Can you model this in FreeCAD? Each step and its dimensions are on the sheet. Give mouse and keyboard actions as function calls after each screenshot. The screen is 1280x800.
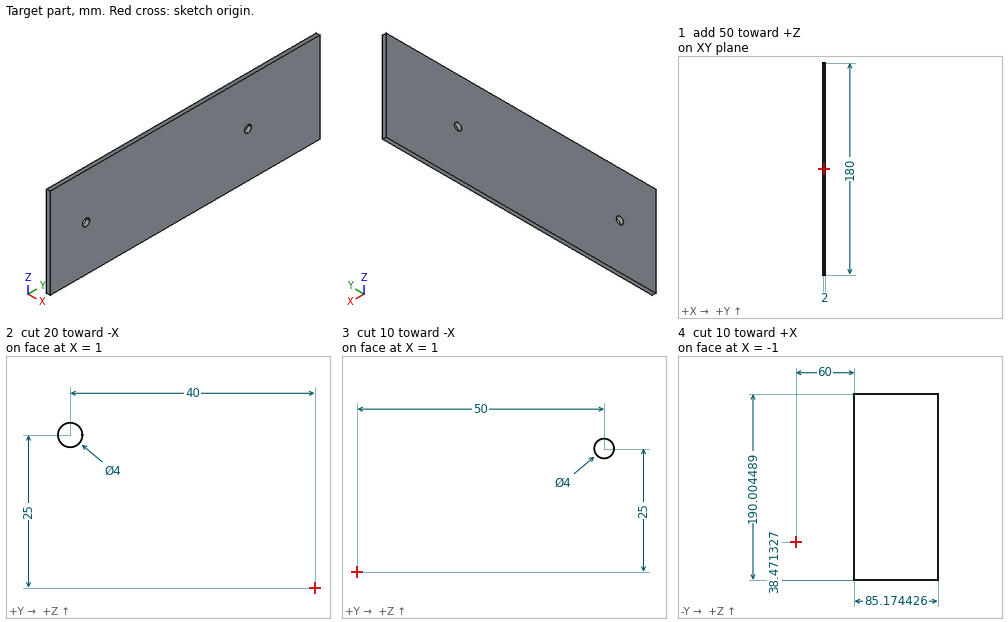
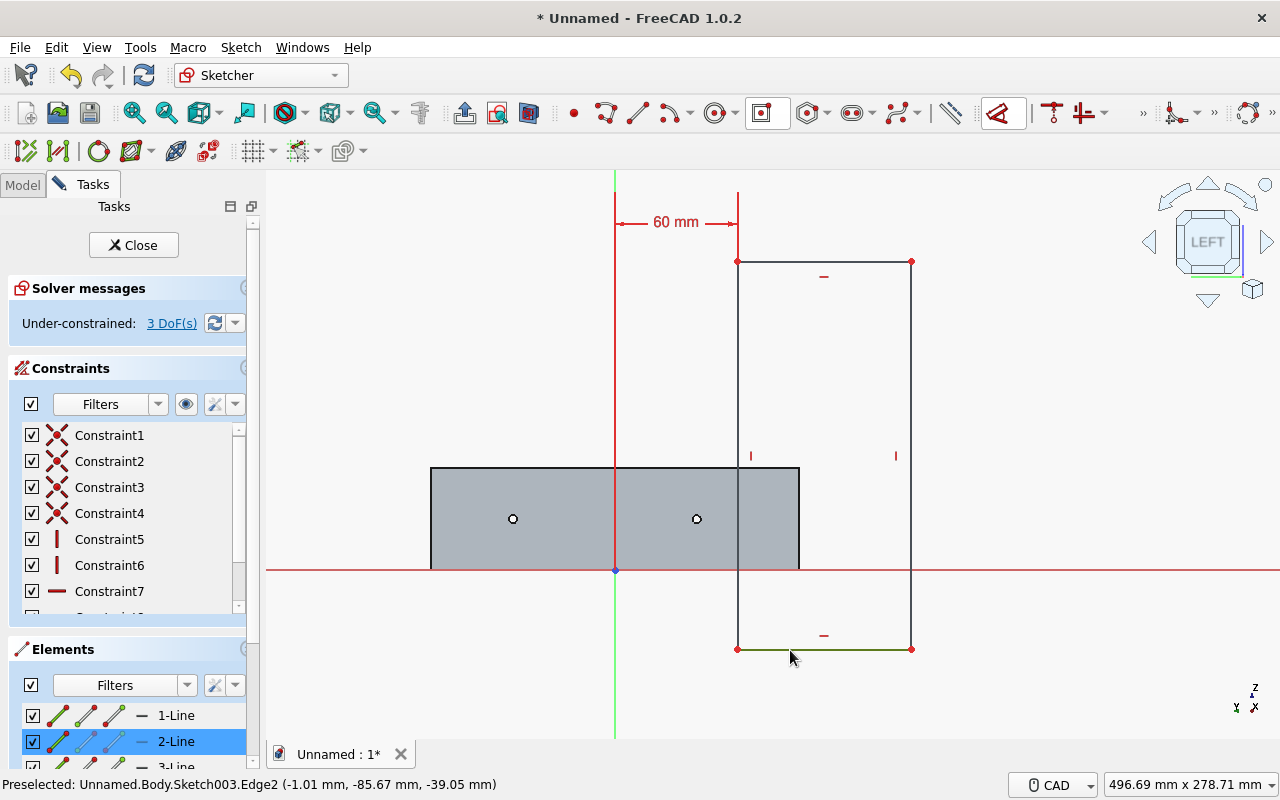
click(1020, 114)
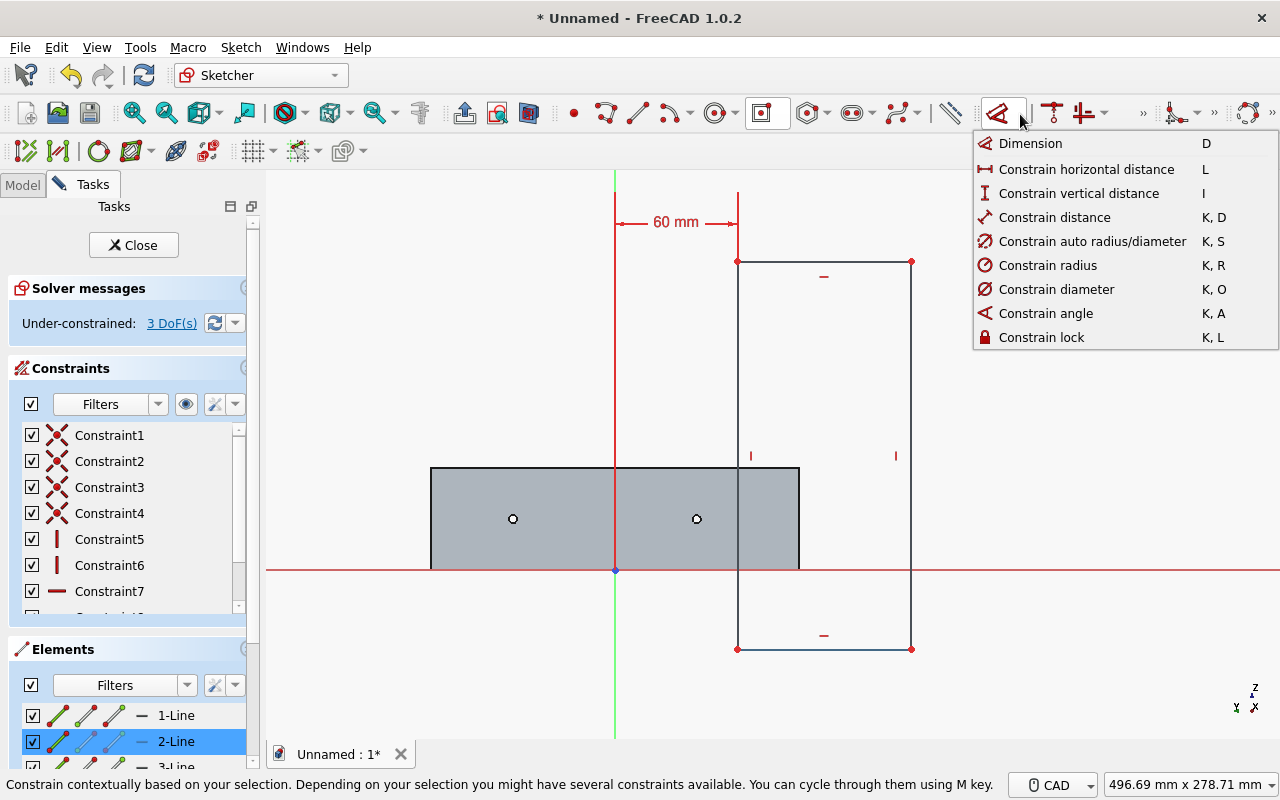
click(1126, 169)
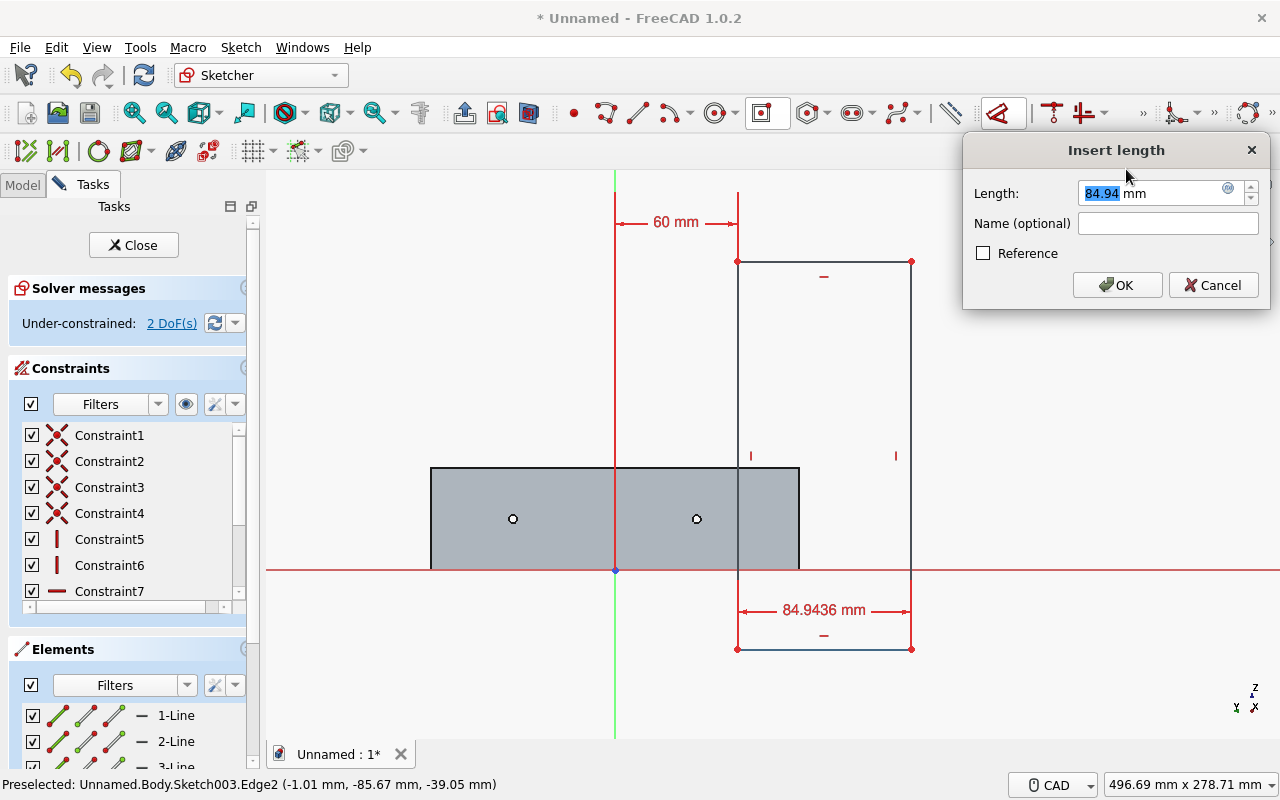
text(85.174426)
key(Return)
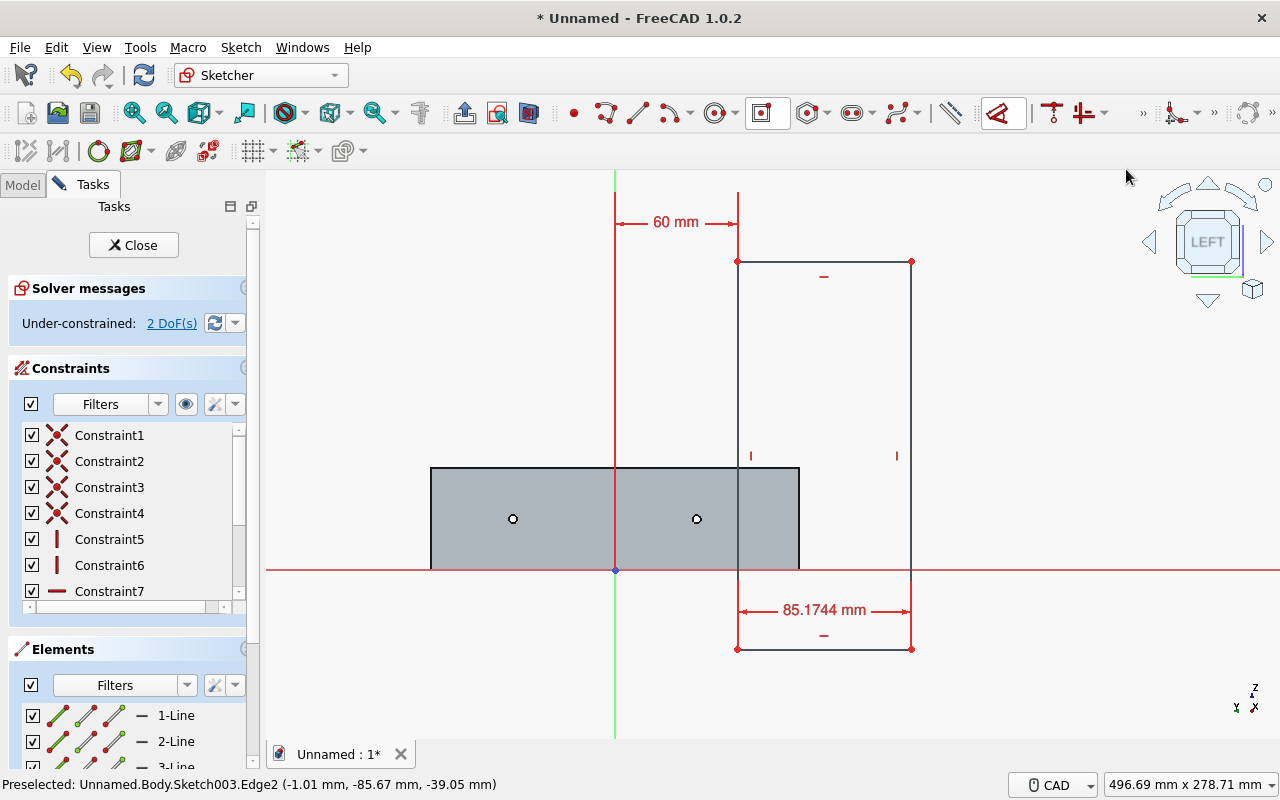
click(738, 378)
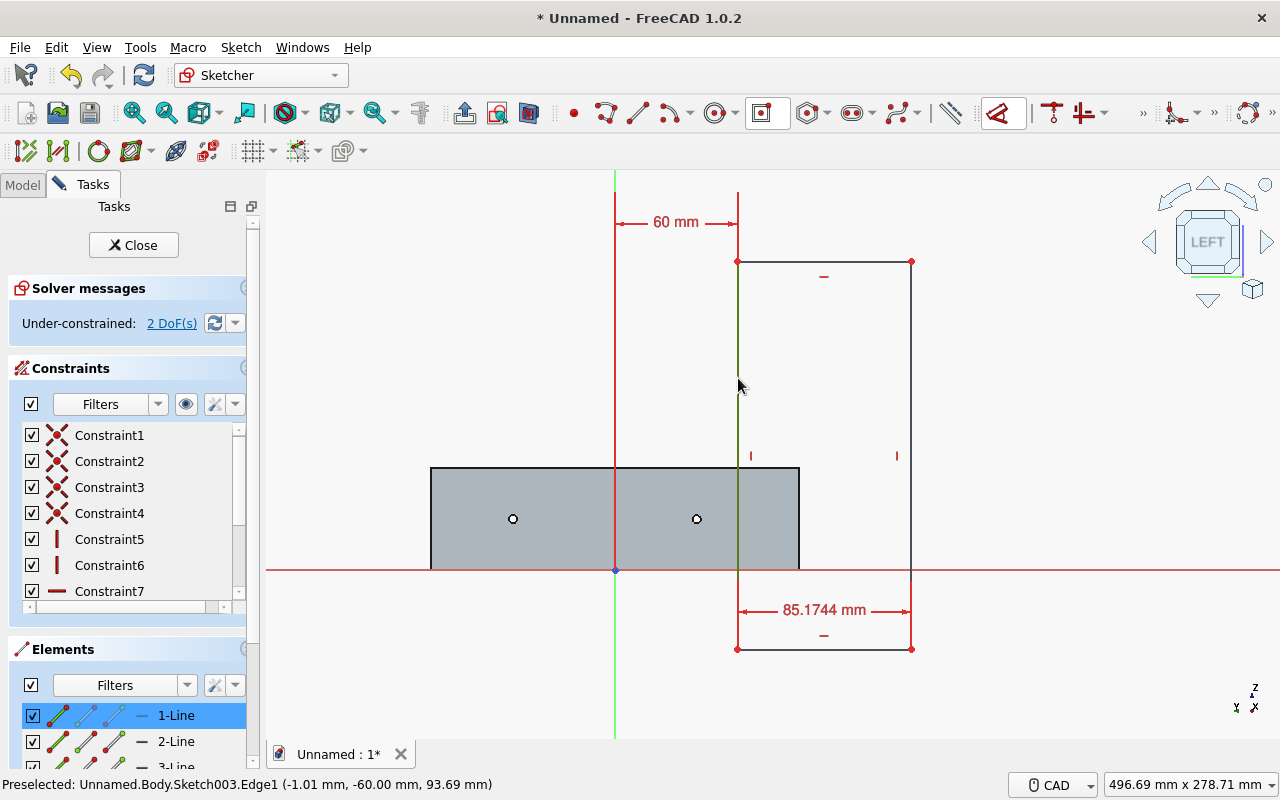
click(1020, 114)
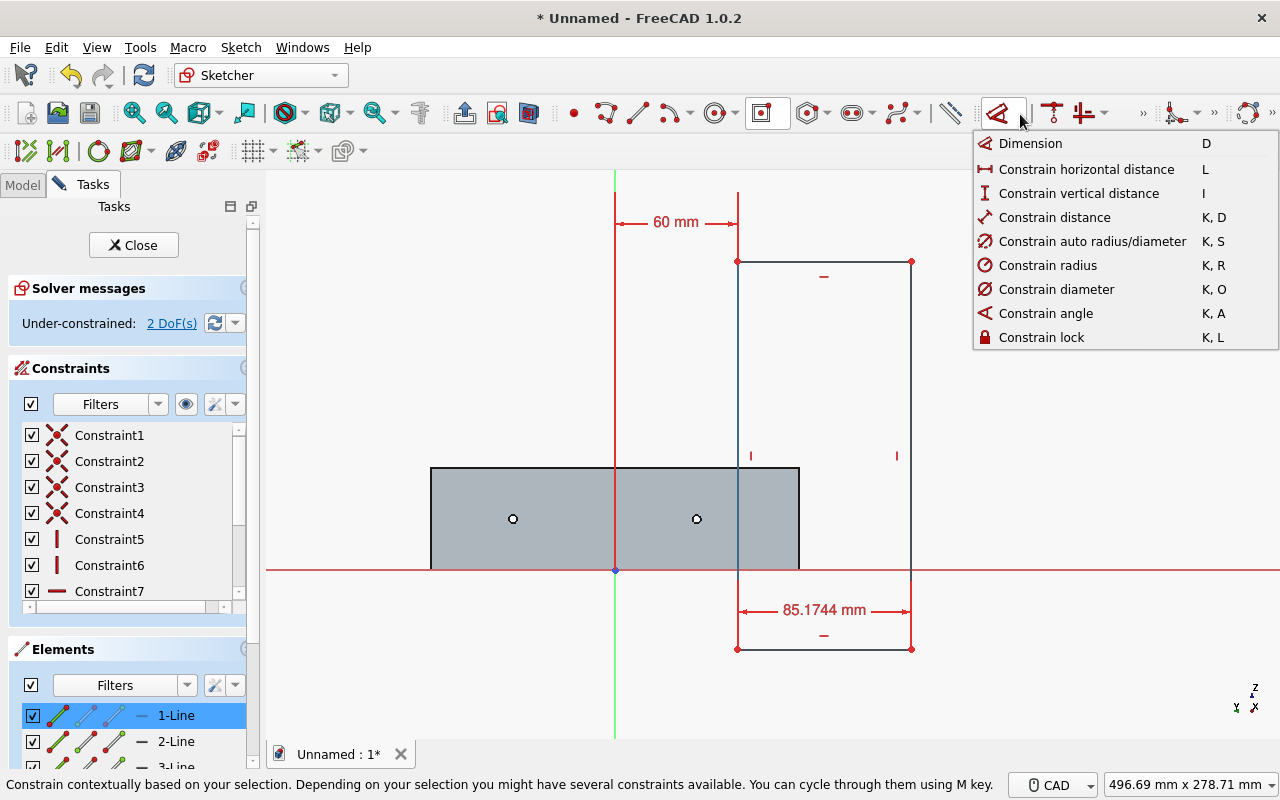
click(1126, 193)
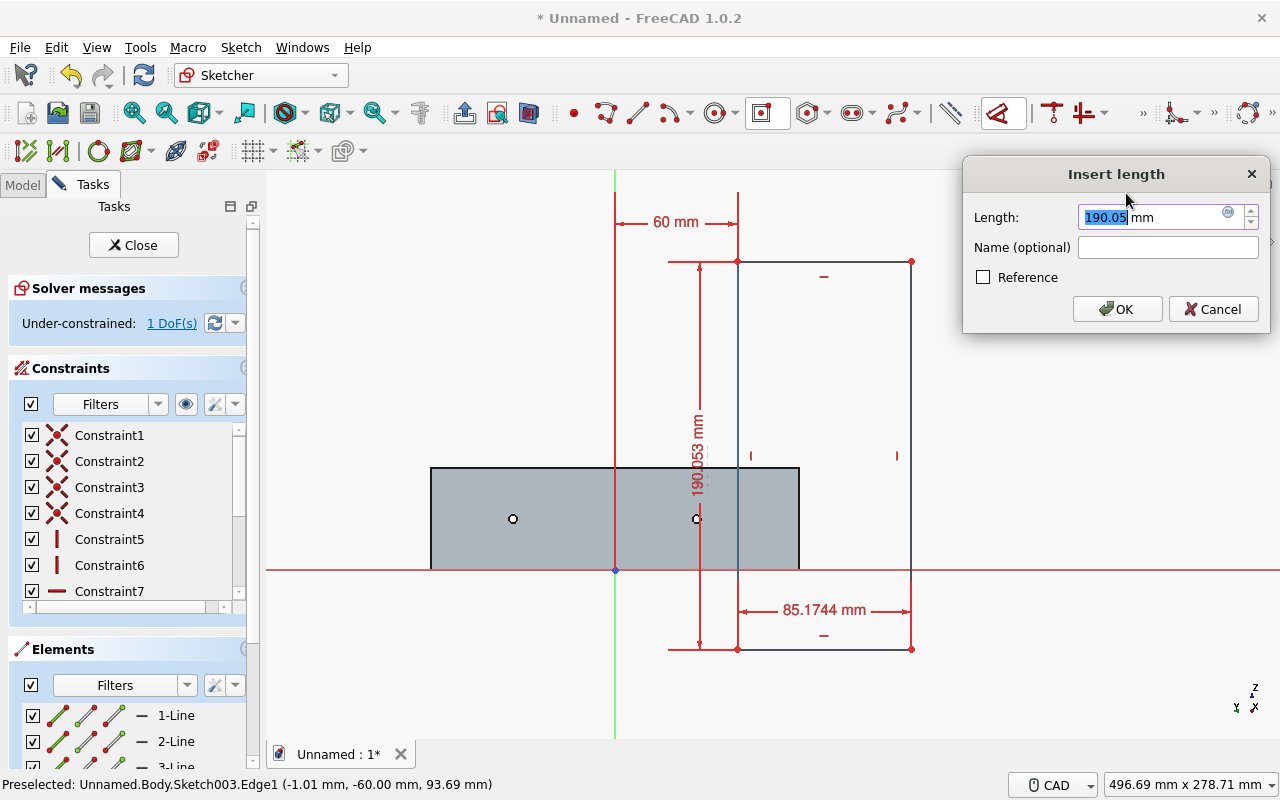
text(190.004489)
key(Return)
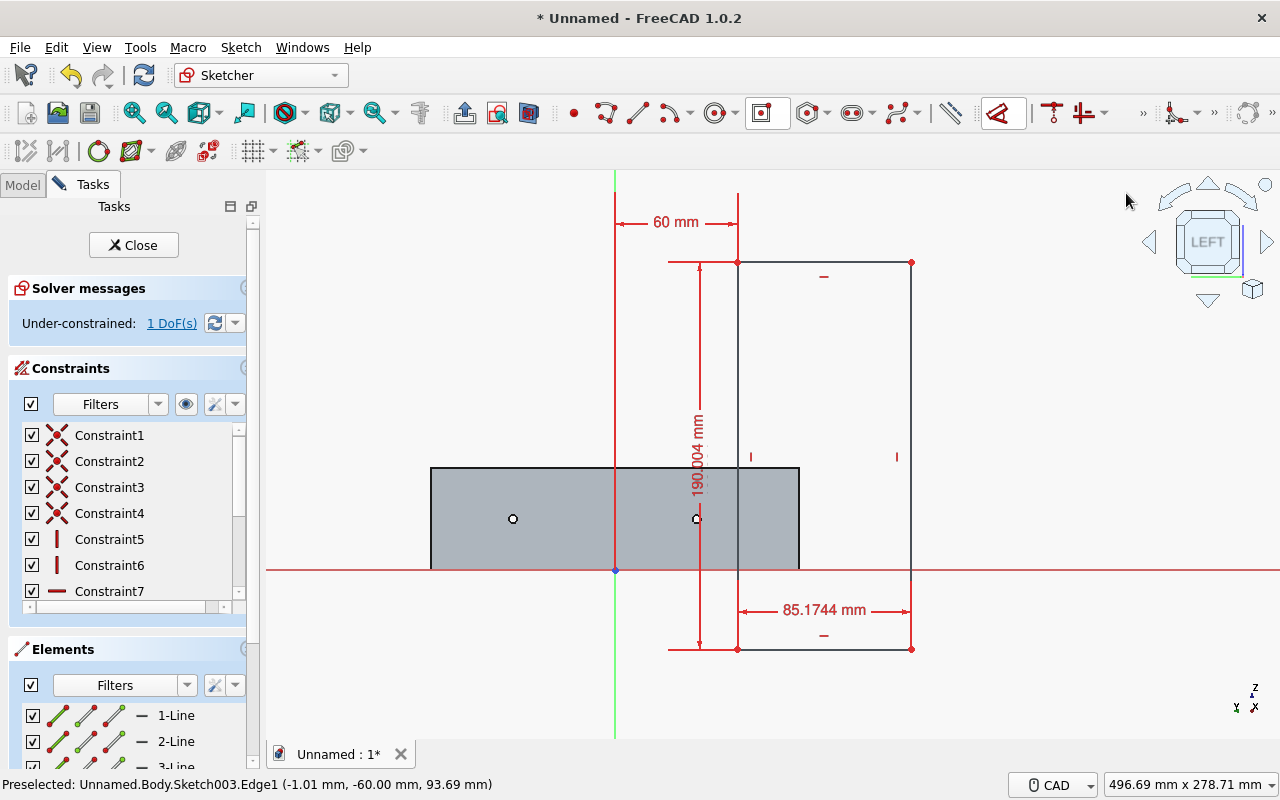
click(738, 650)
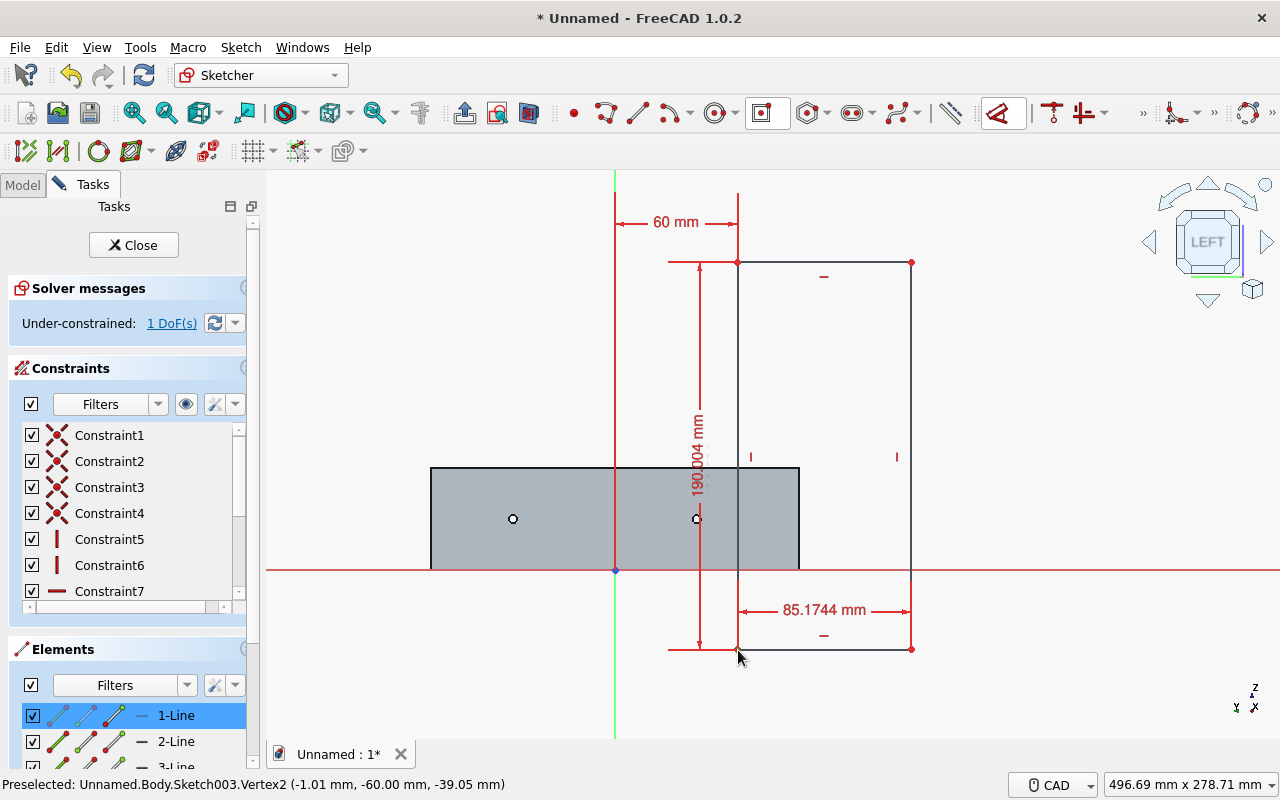
click(1020, 114)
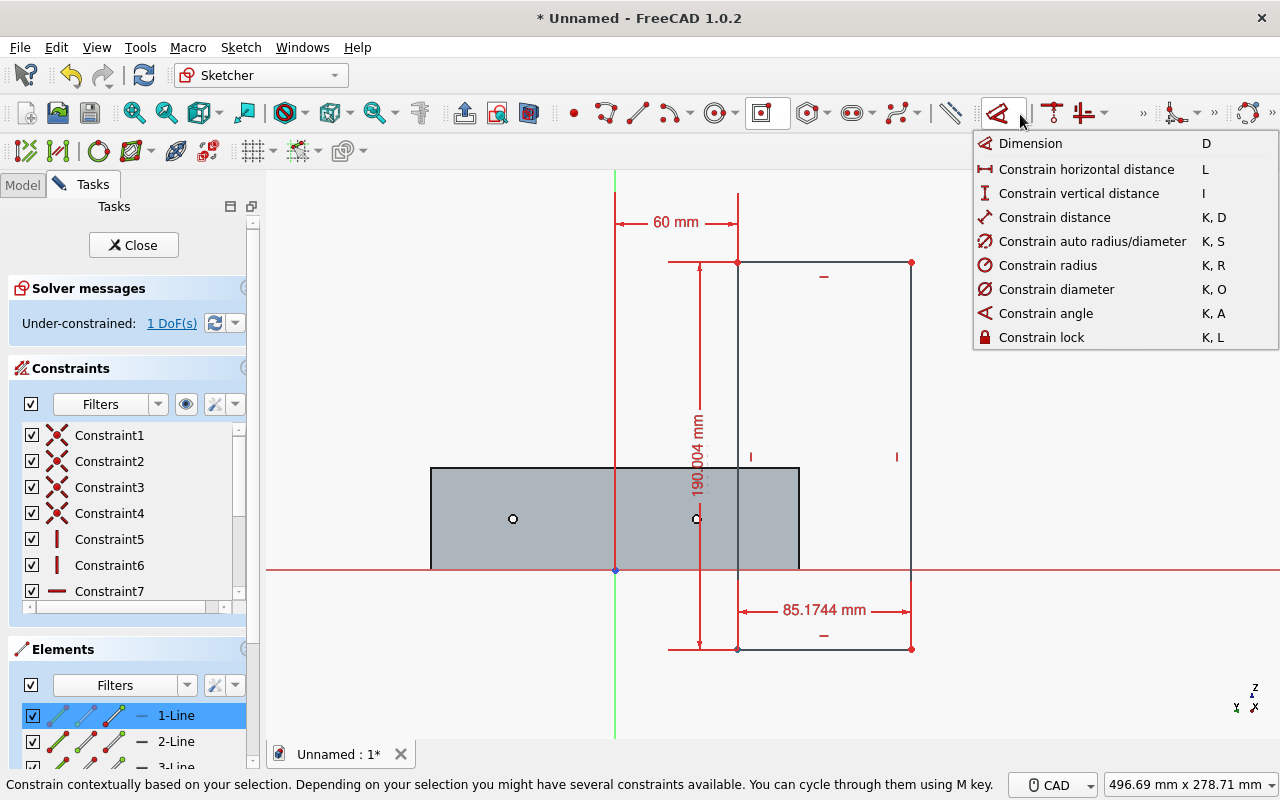
click(1126, 193)